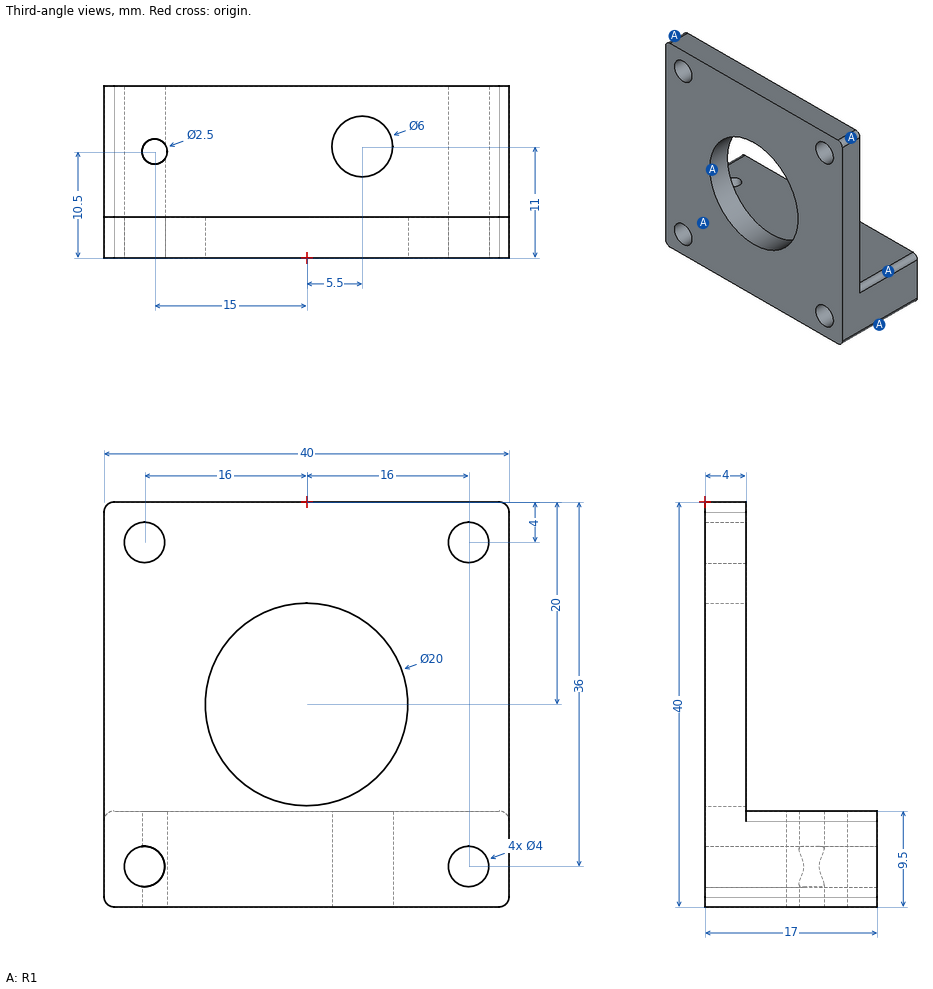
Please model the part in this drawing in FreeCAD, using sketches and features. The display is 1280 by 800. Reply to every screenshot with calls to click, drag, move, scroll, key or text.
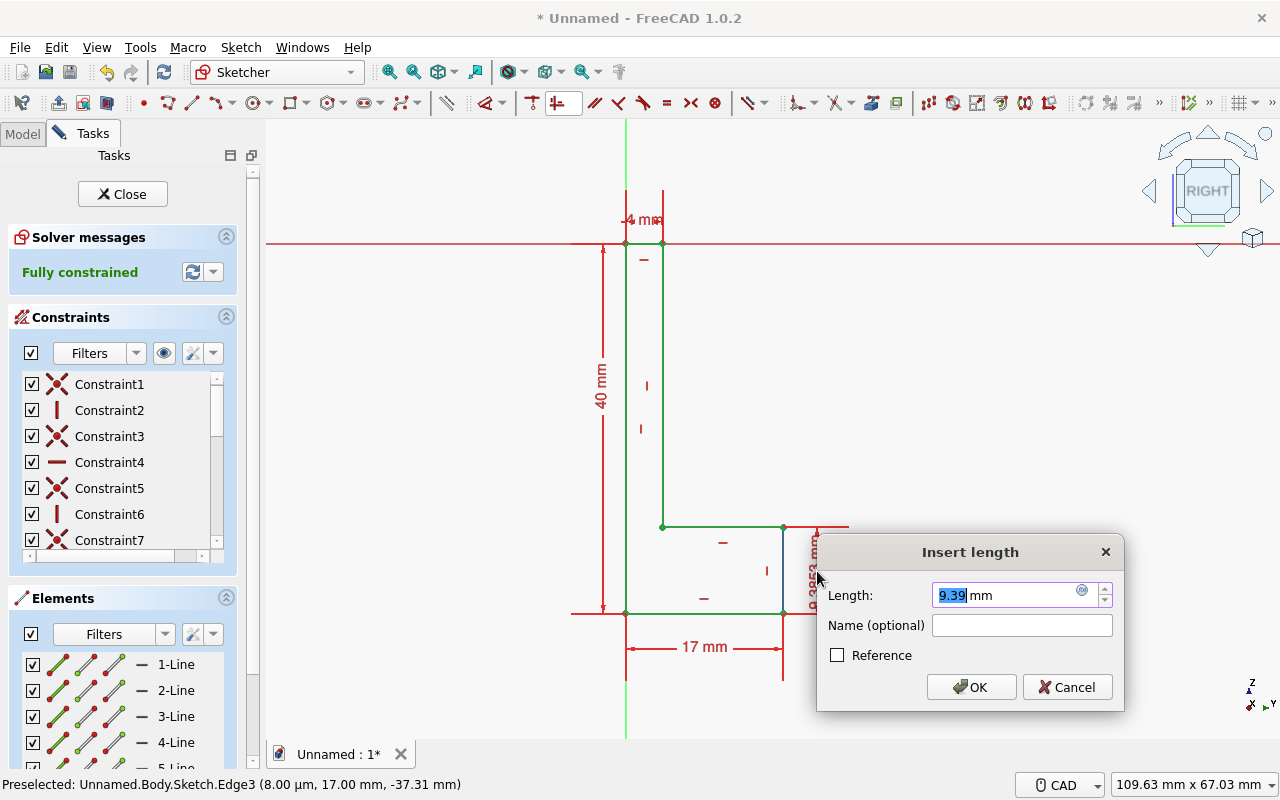
text(9.5)
key(Return)
key(Escape)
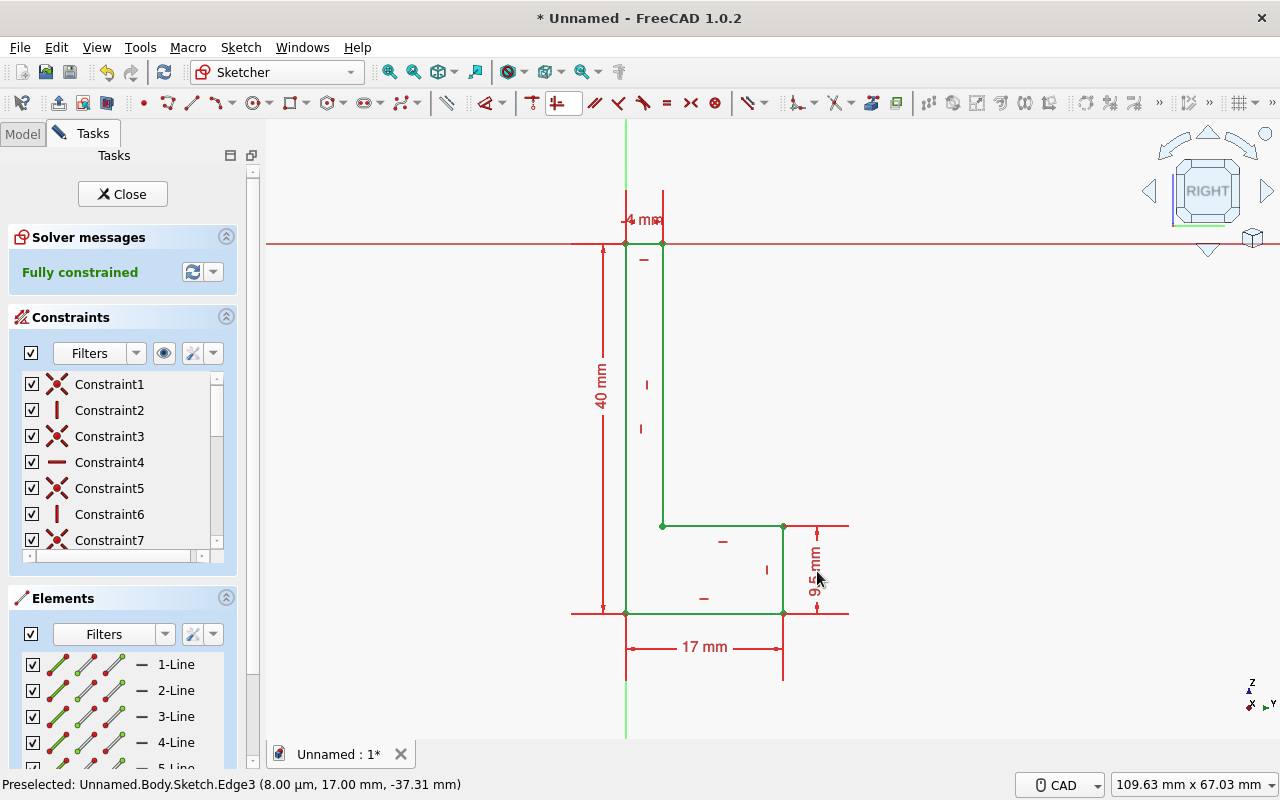
click(123, 194)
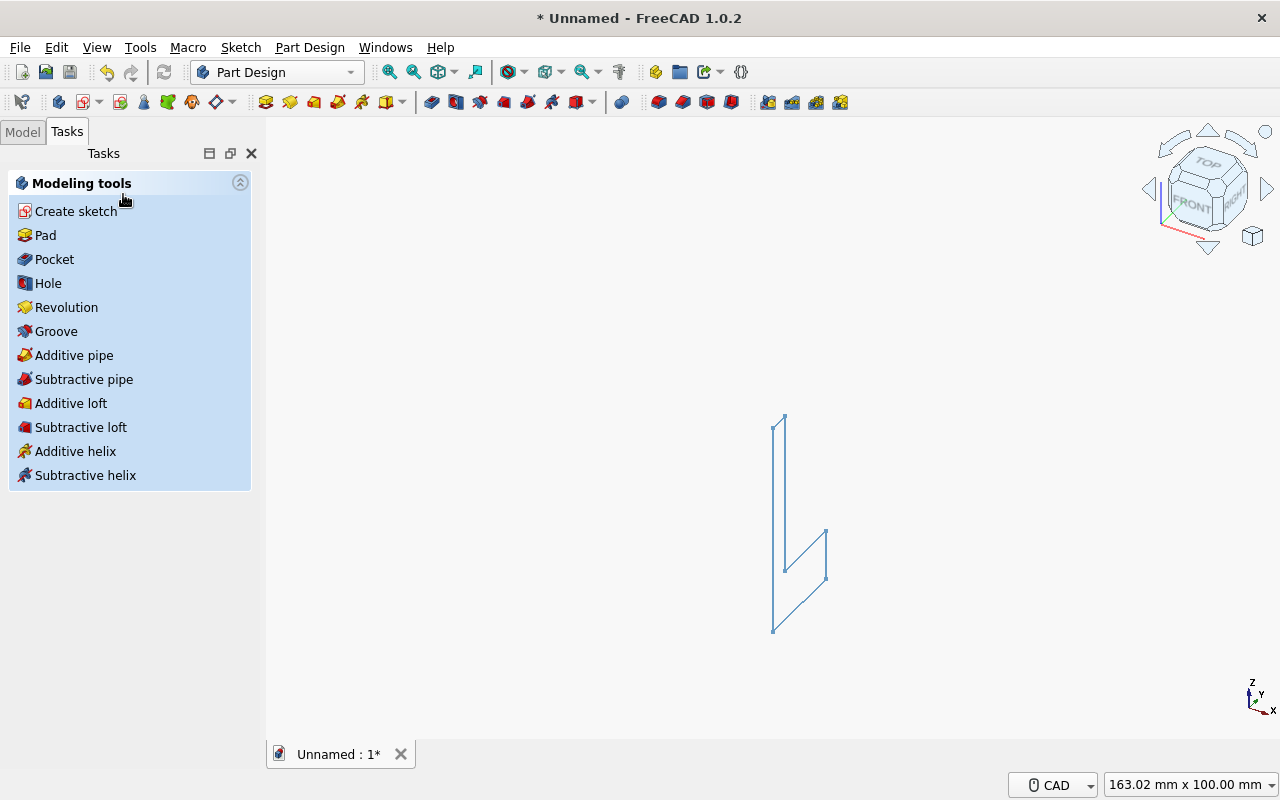
click(266, 102)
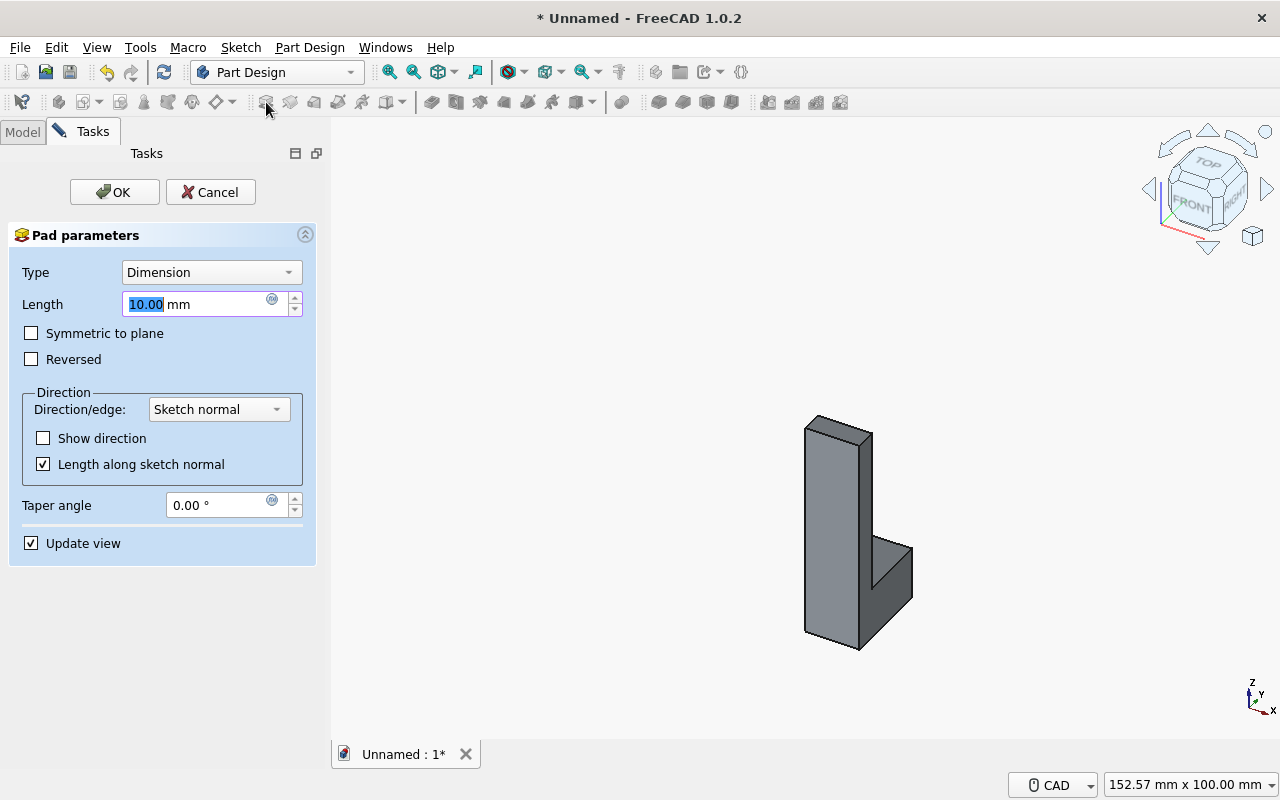
text(40)
key(Tab)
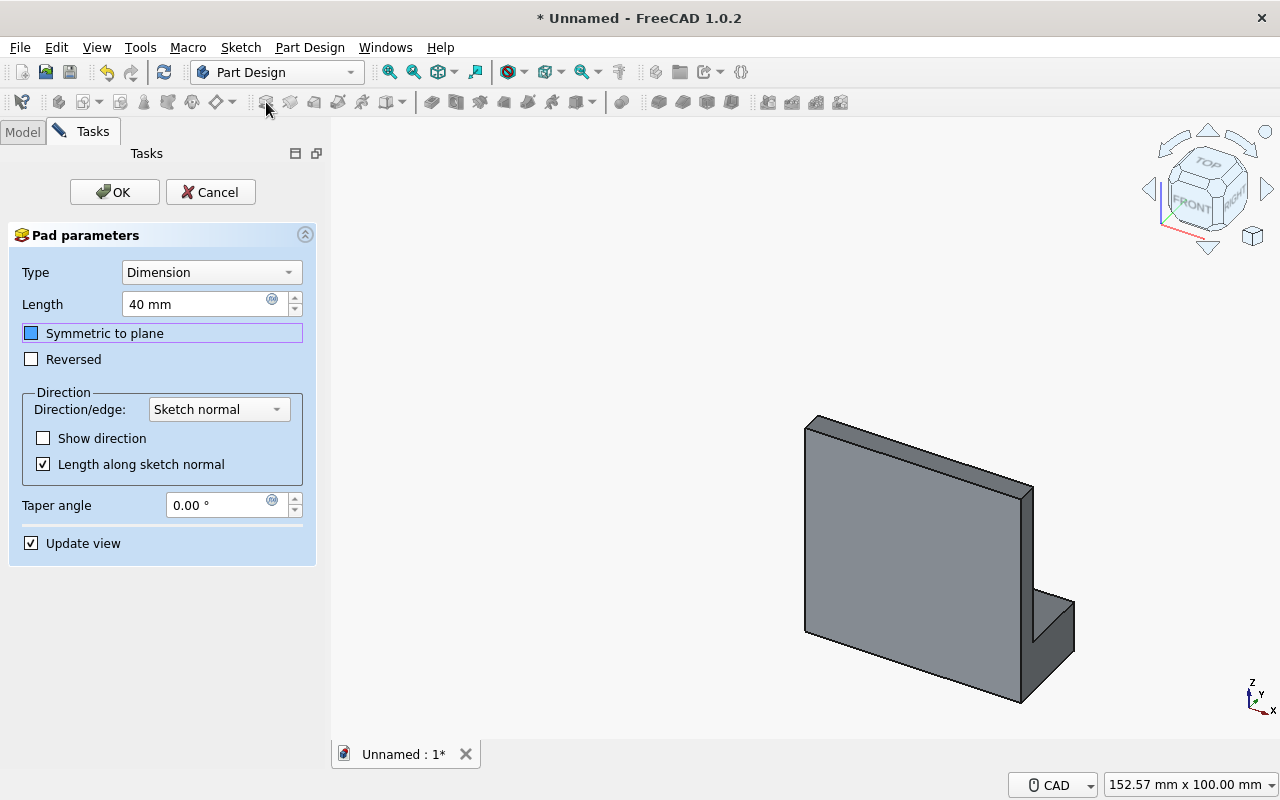
click(30, 333)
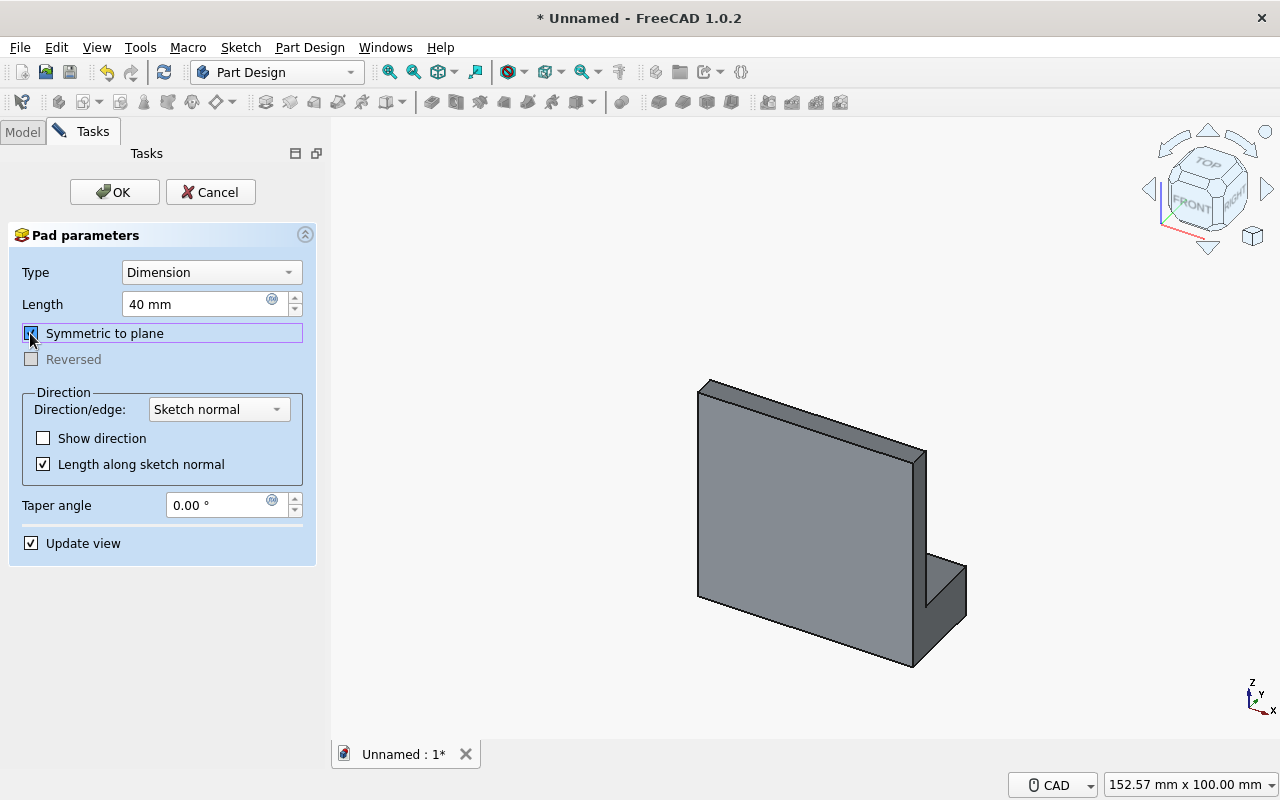
click(115, 192)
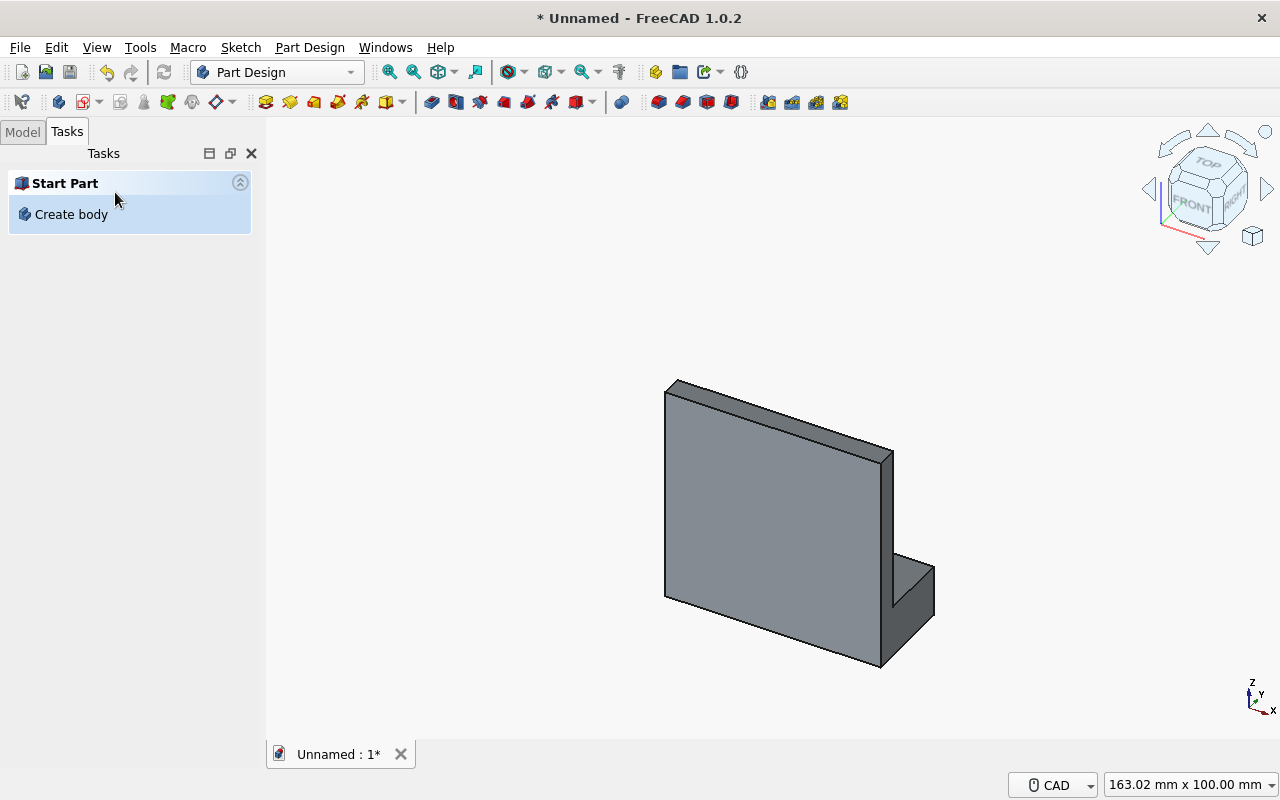
key(4)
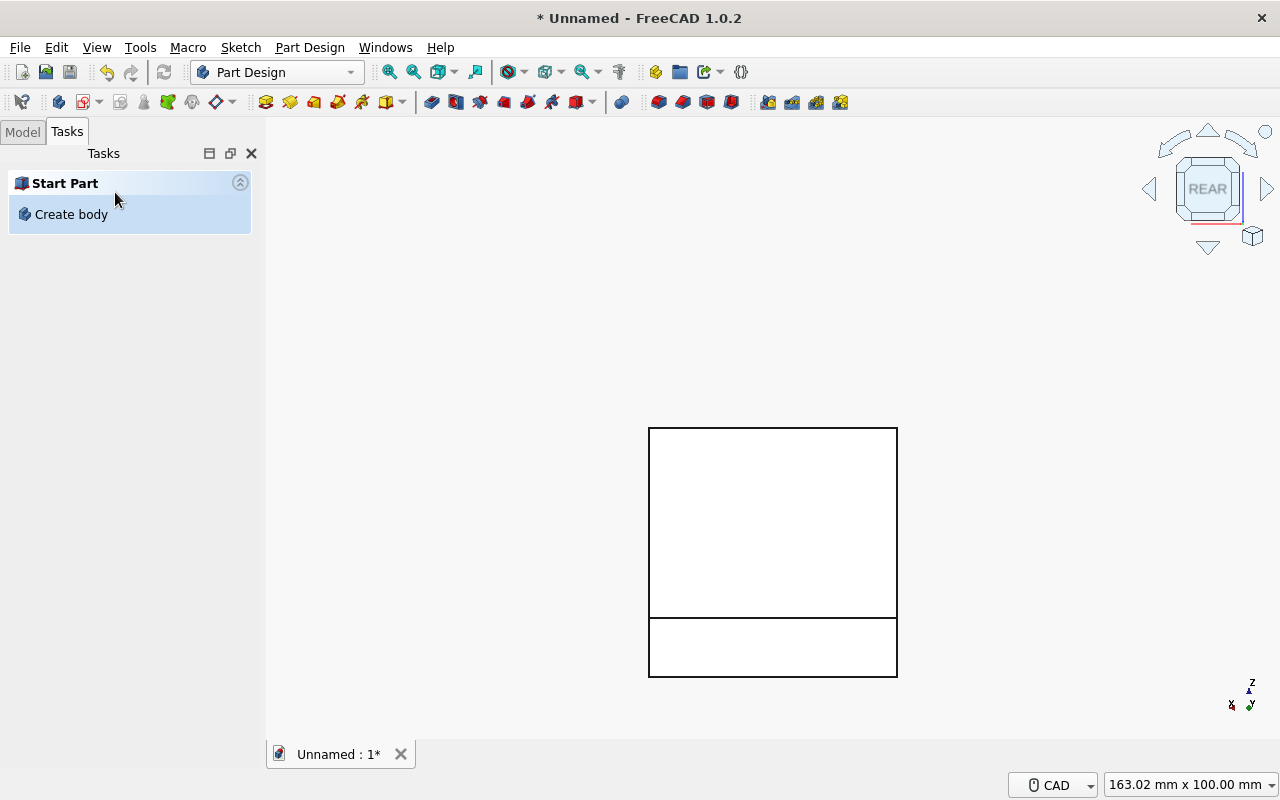
click(390, 72)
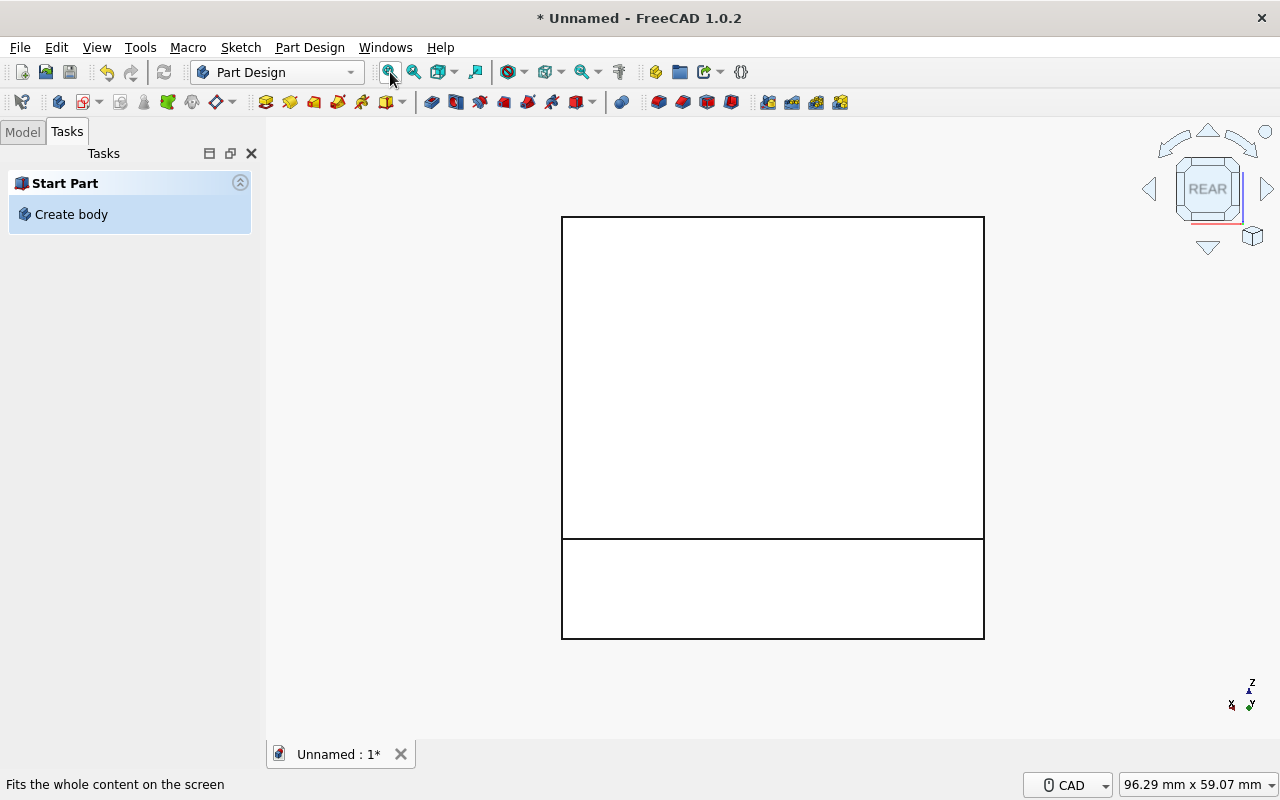
click(773, 377)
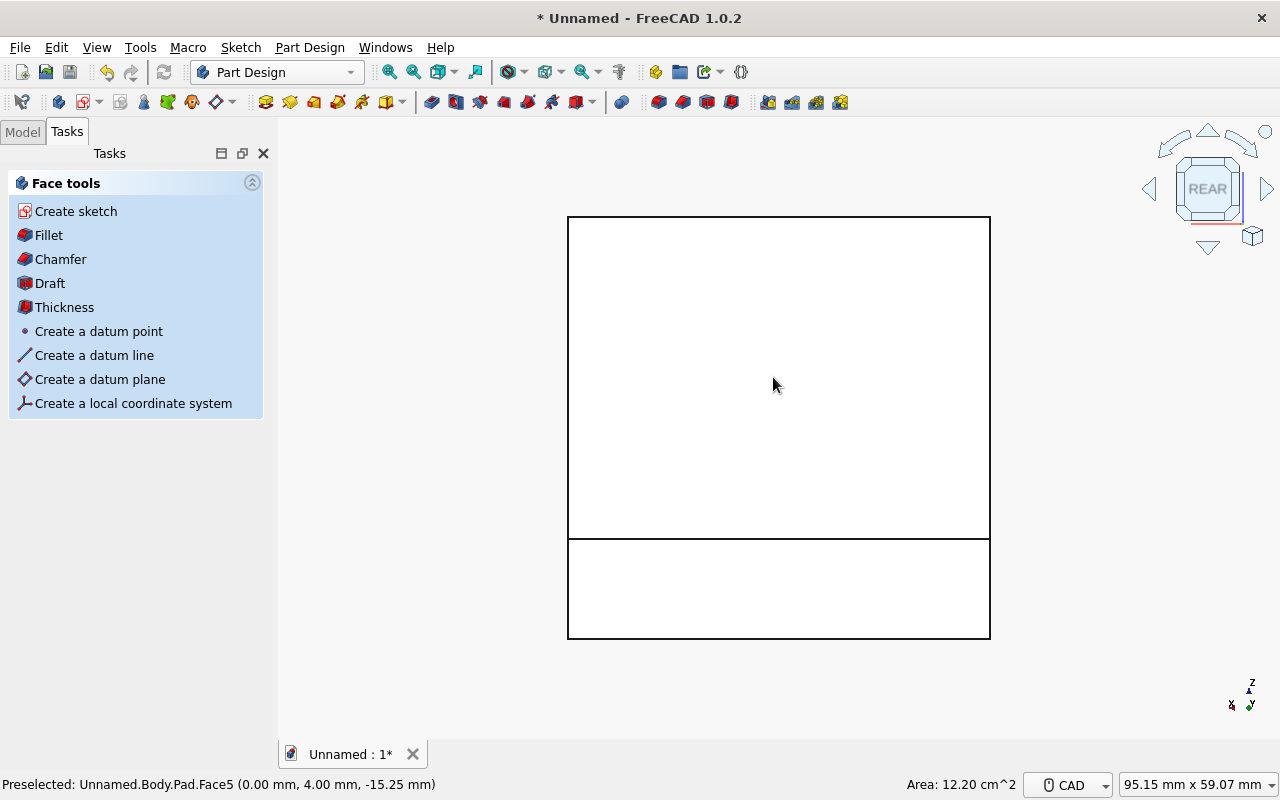
click(84, 102)